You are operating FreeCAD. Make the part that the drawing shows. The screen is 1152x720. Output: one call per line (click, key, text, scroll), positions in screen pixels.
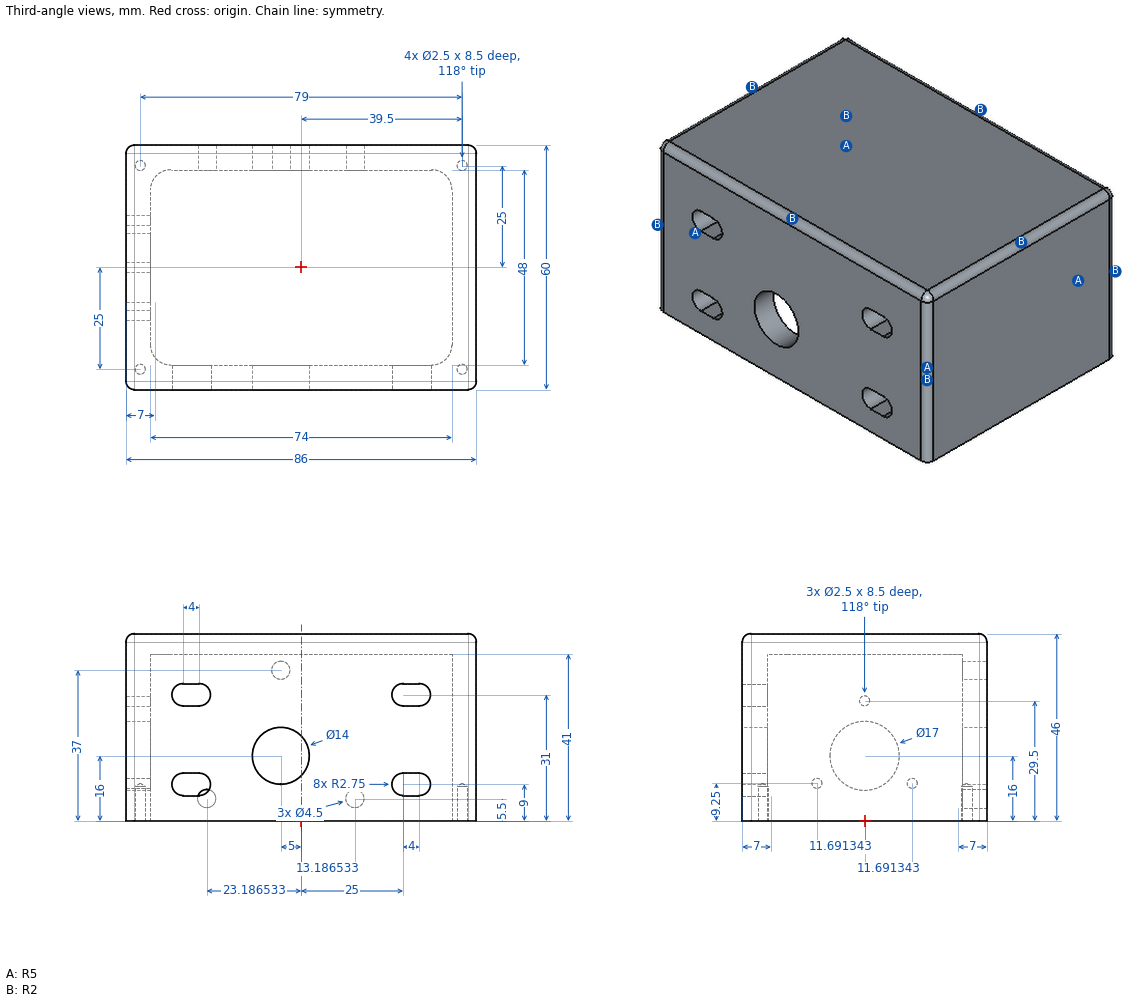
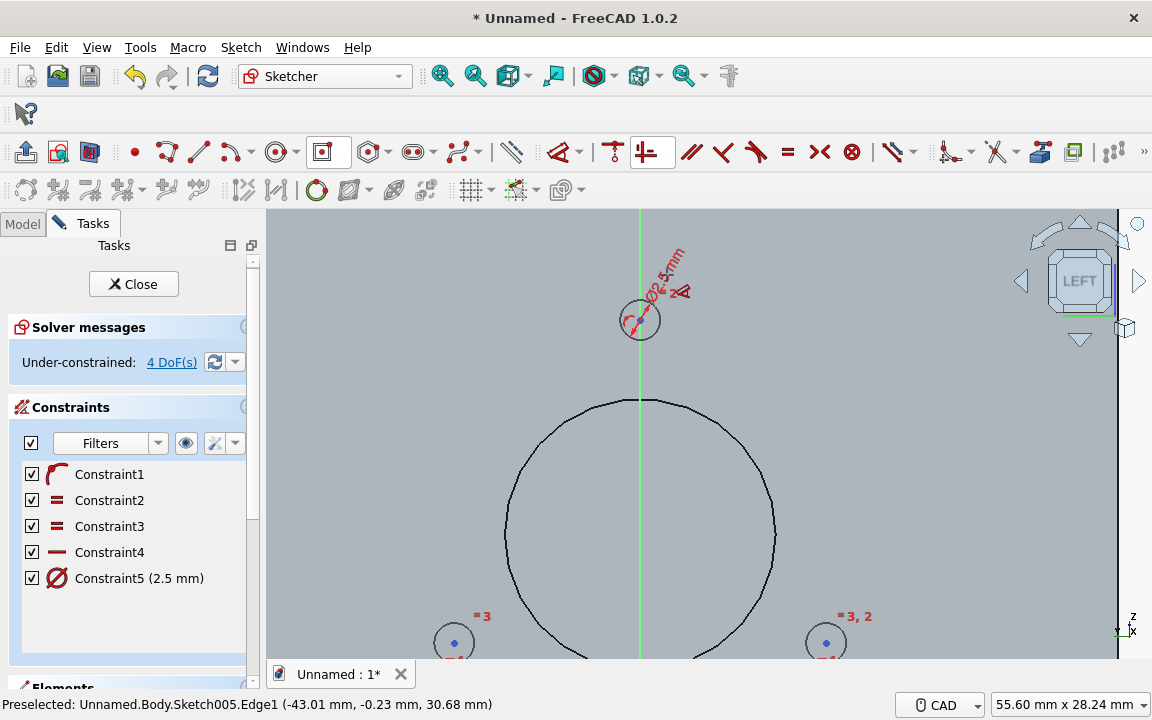
click(640, 320)
click(674, 476)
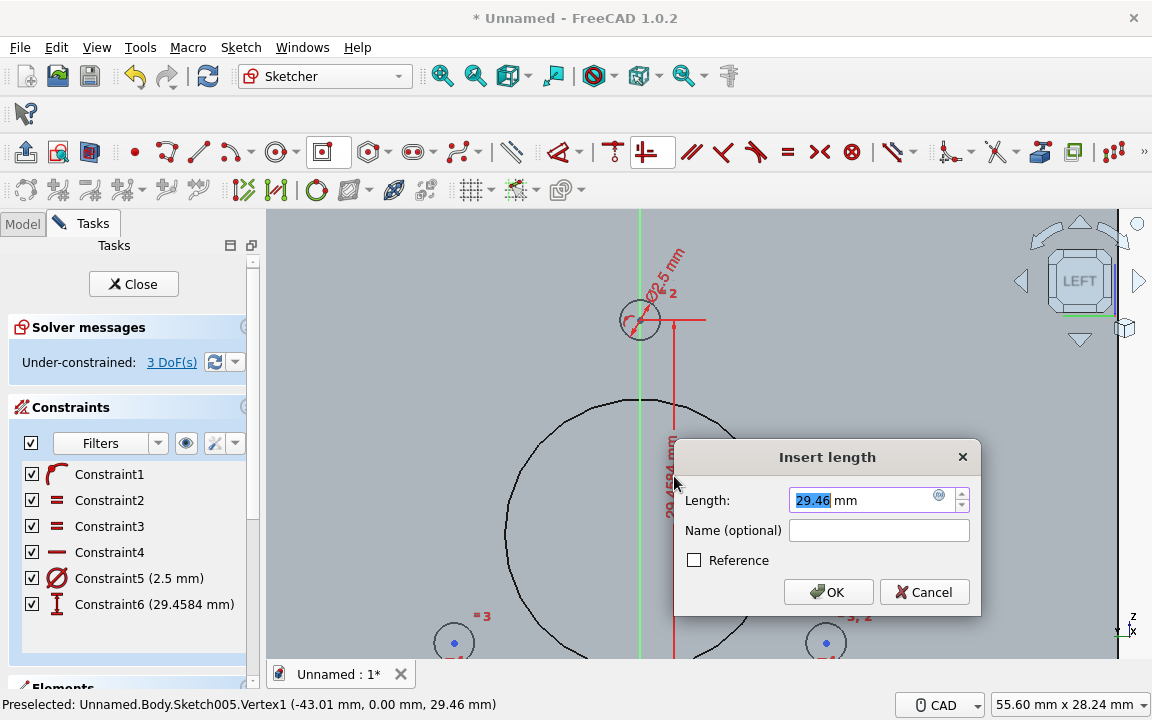
text(29.5)
key(Return)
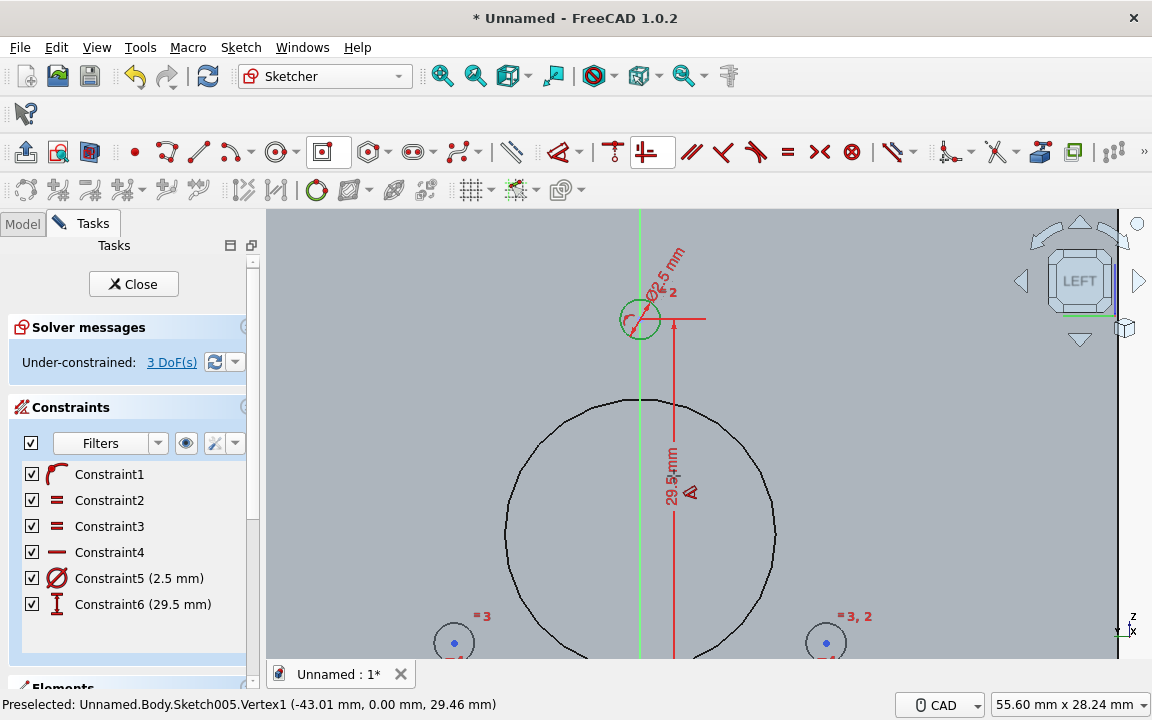
scroll(641, 300, down, 3)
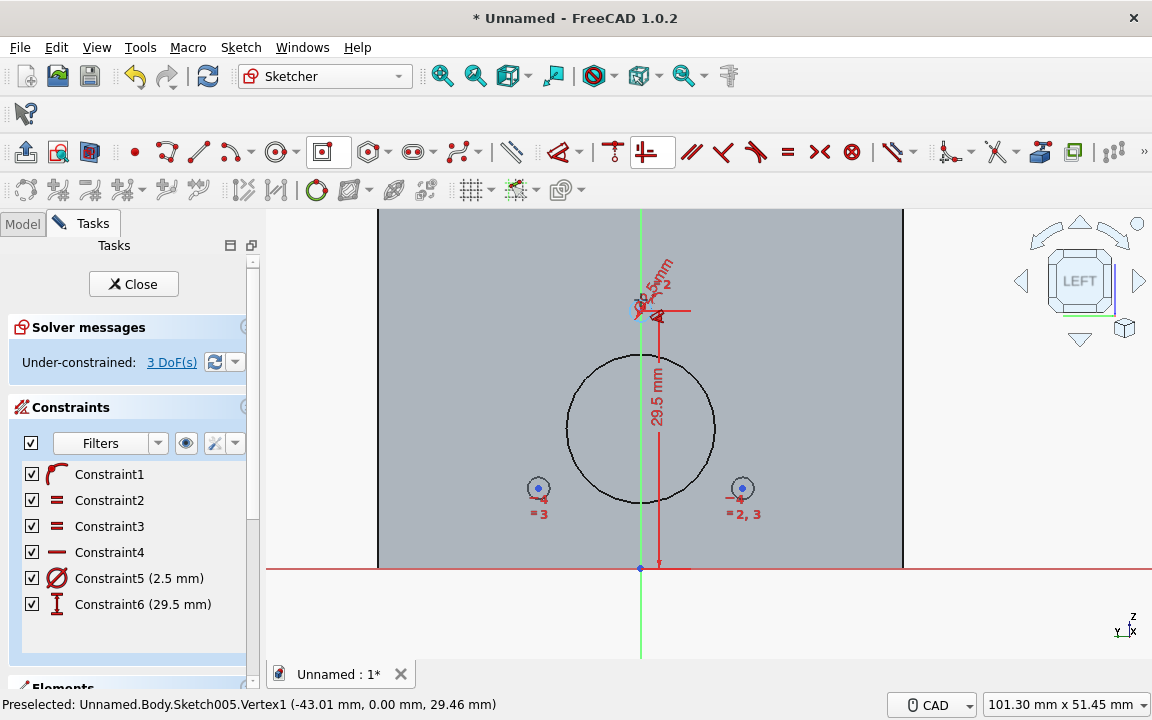
click(743, 488)
click(777, 529)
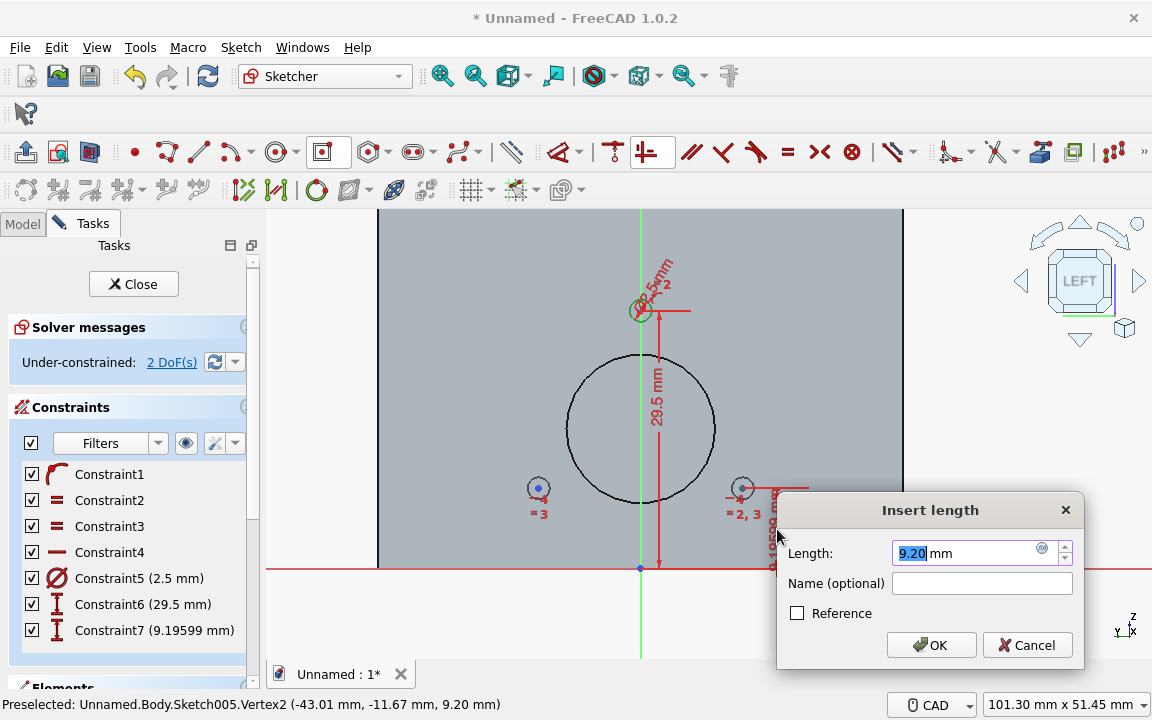
text(9.25)
key(Return)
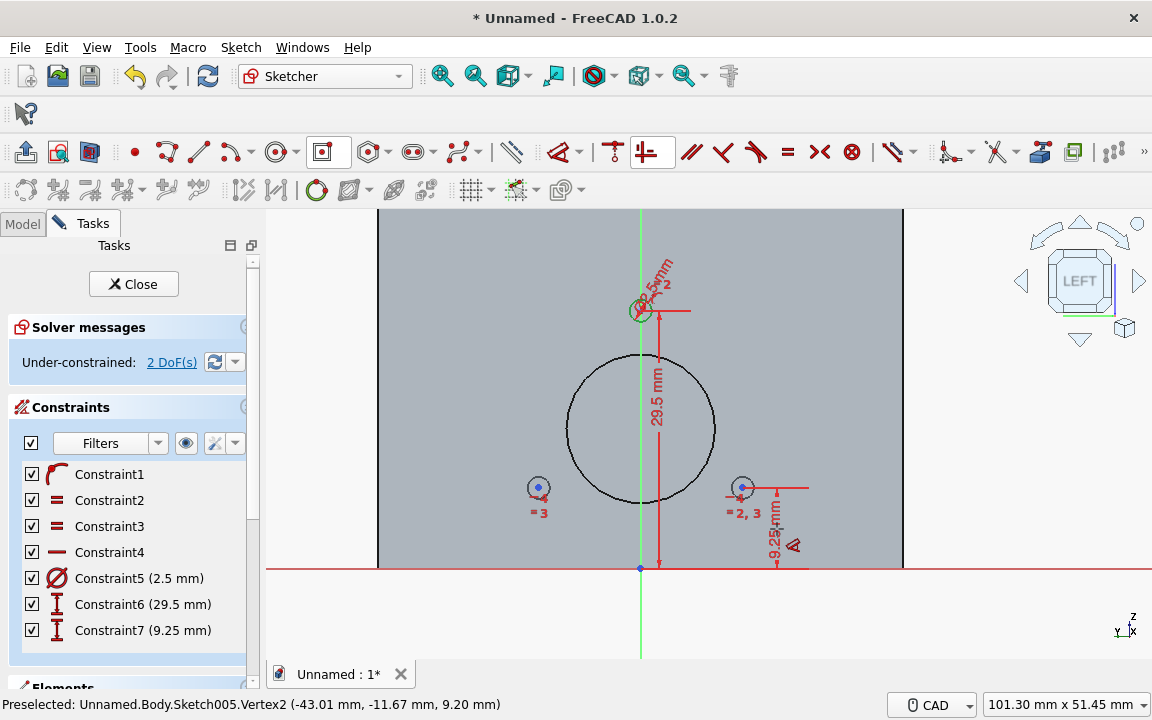
click(743, 488)
click(692, 603)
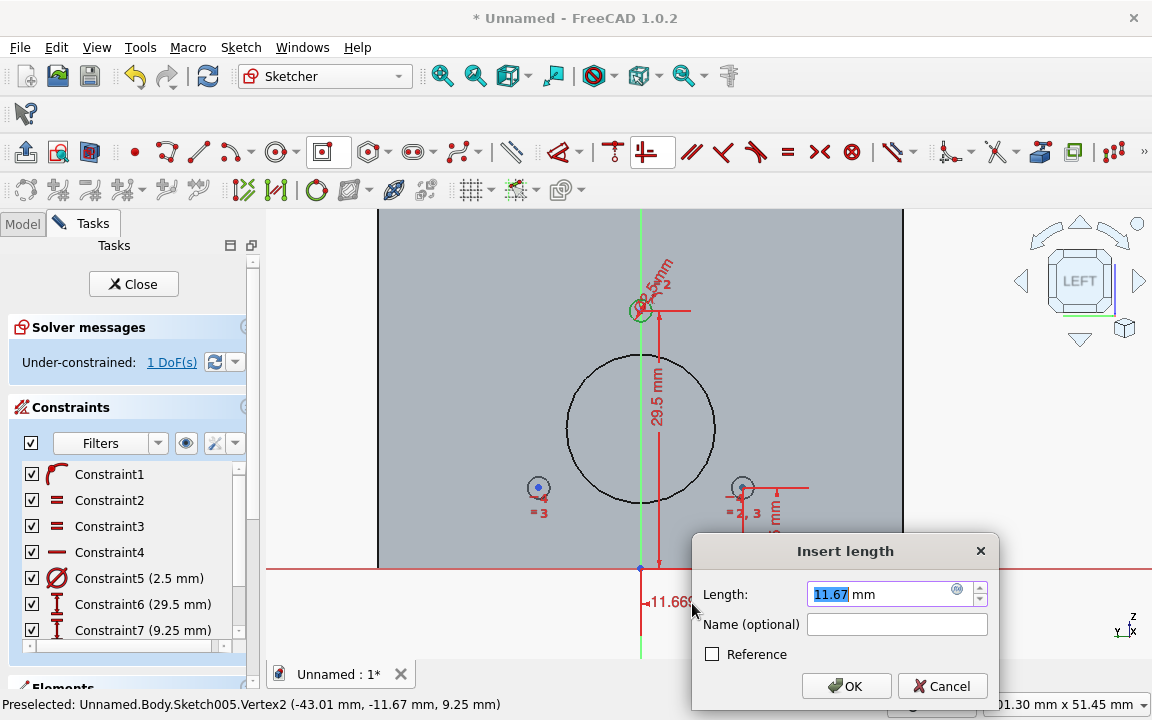
text(11.691343)
key(Return)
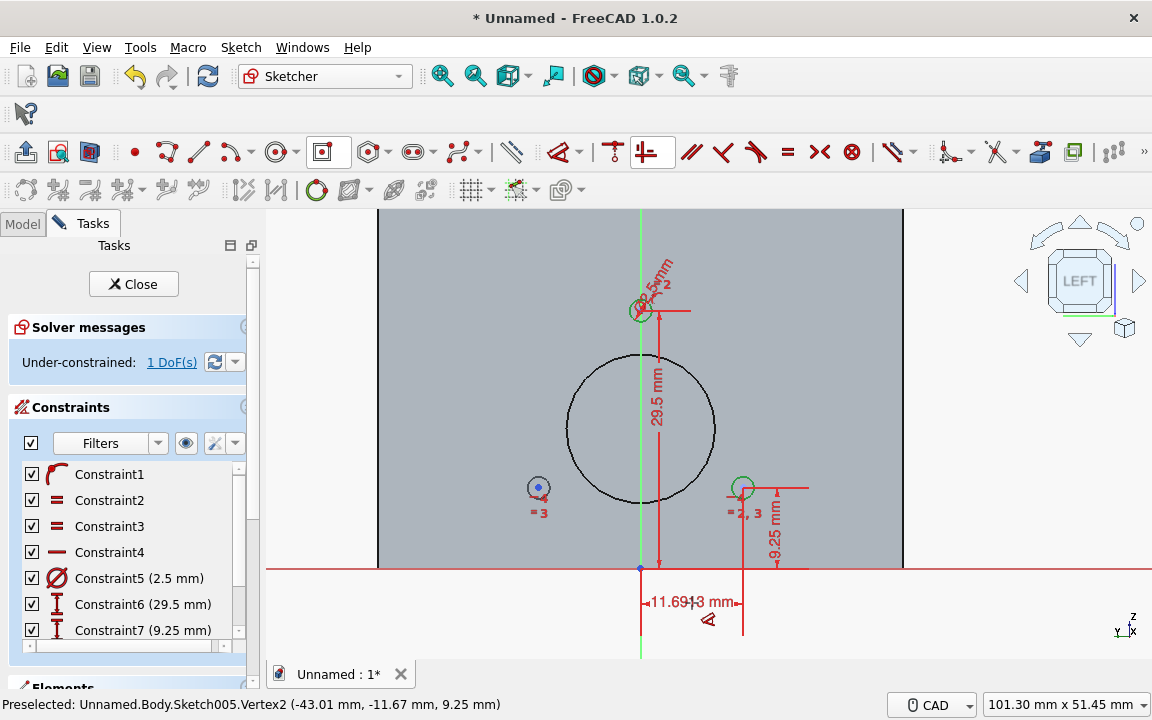
click(539, 488)
click(590, 603)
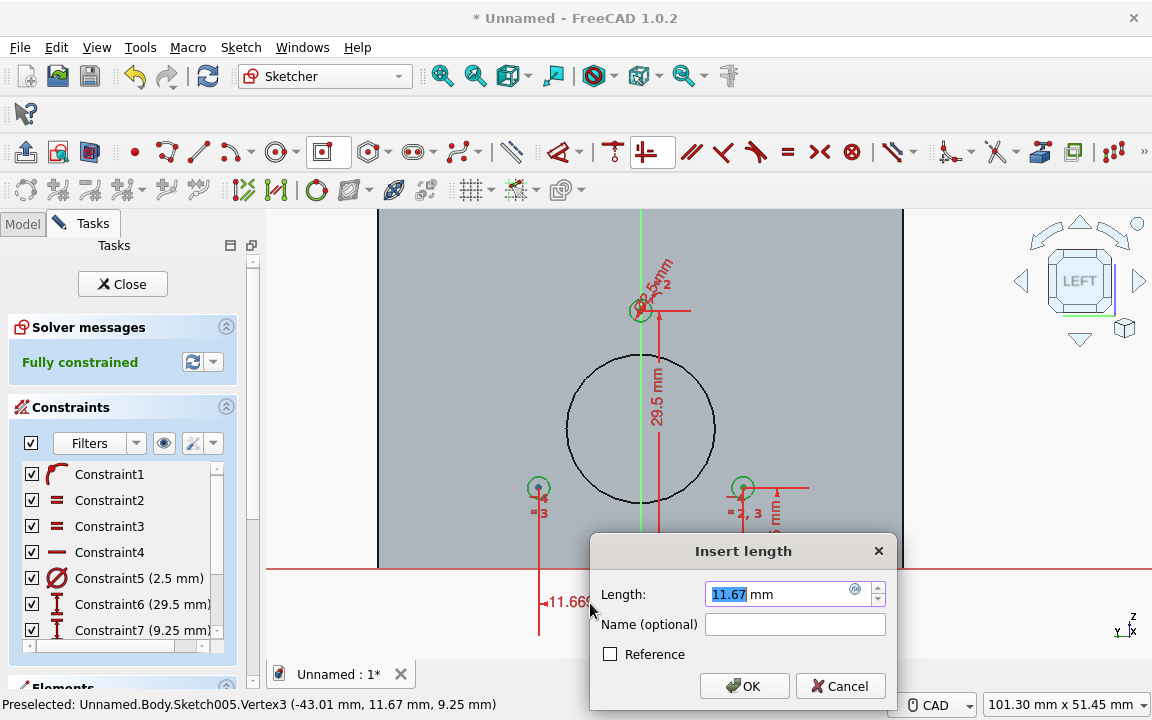
text(11.691343)
key(Return)
key(Escape)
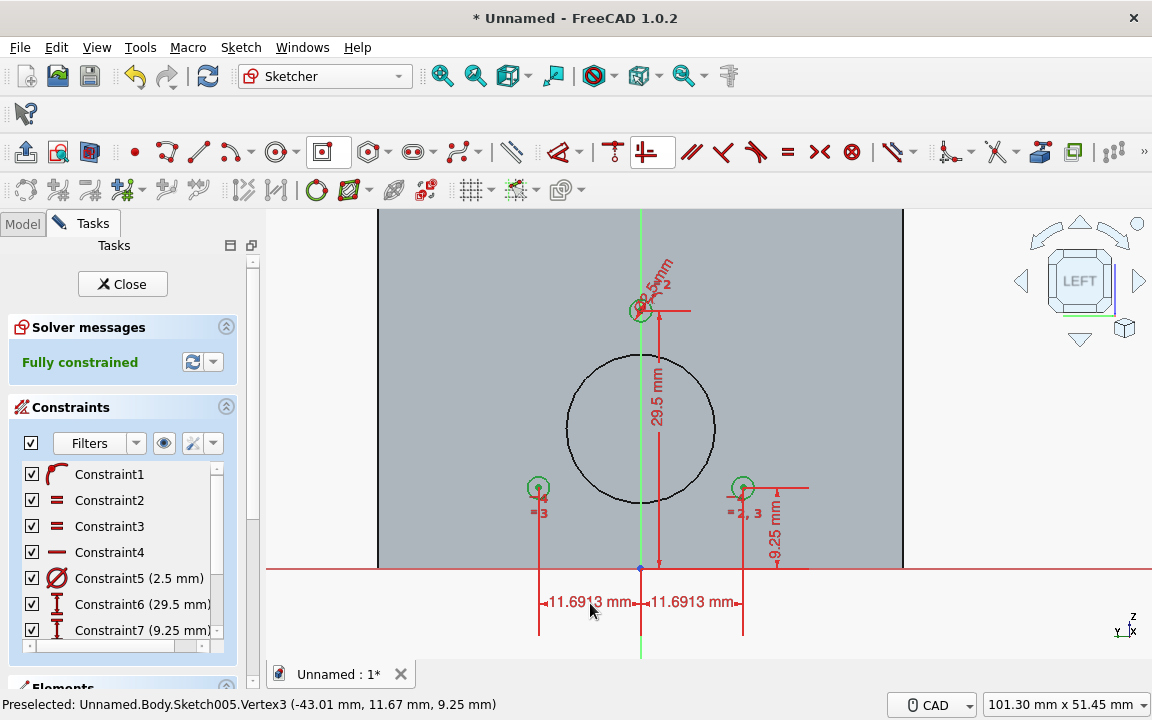
click(123, 284)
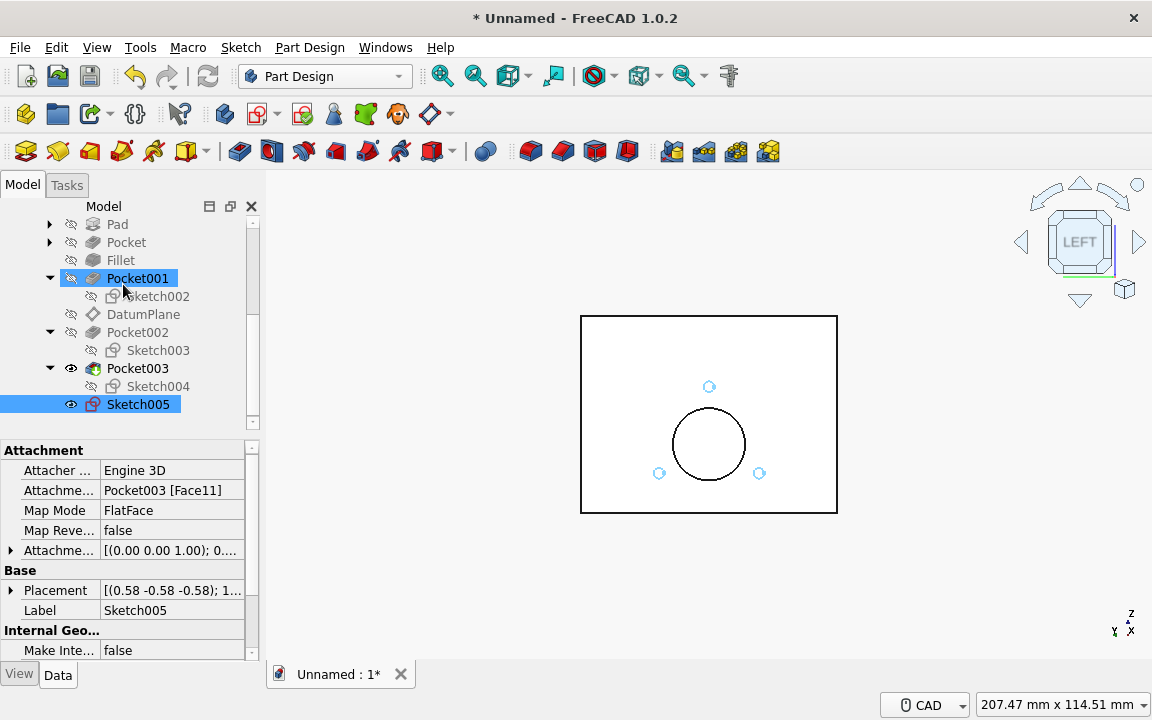
click(272, 152)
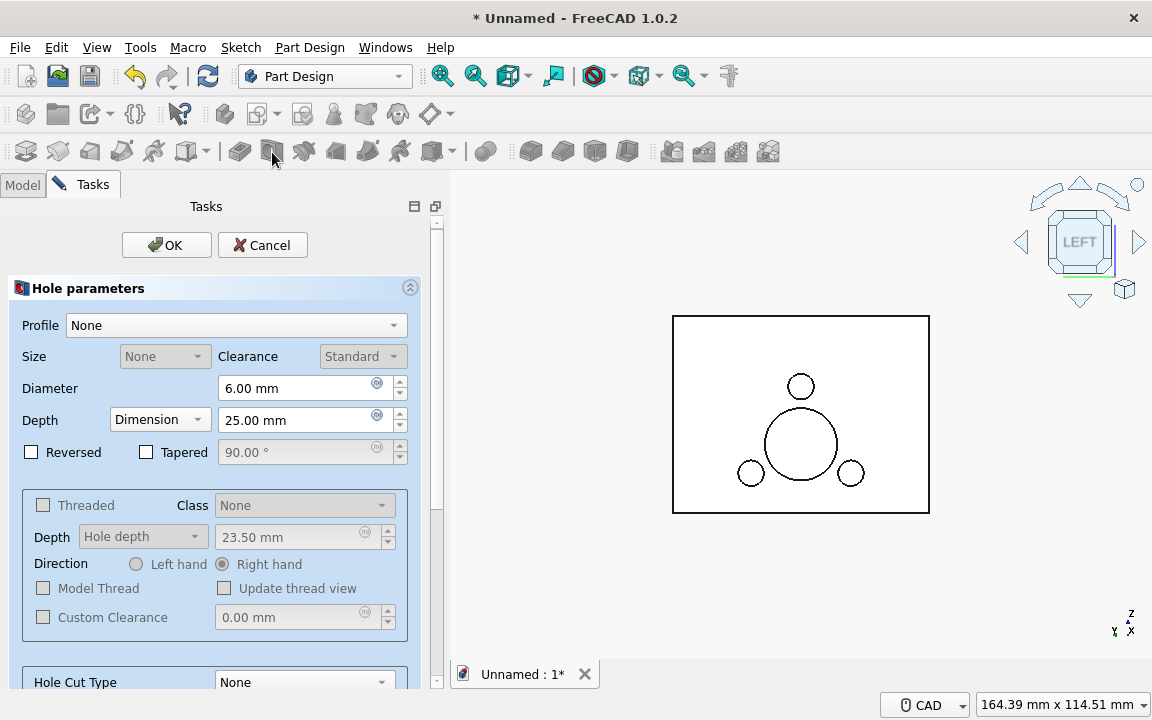
triple_click(305, 388)